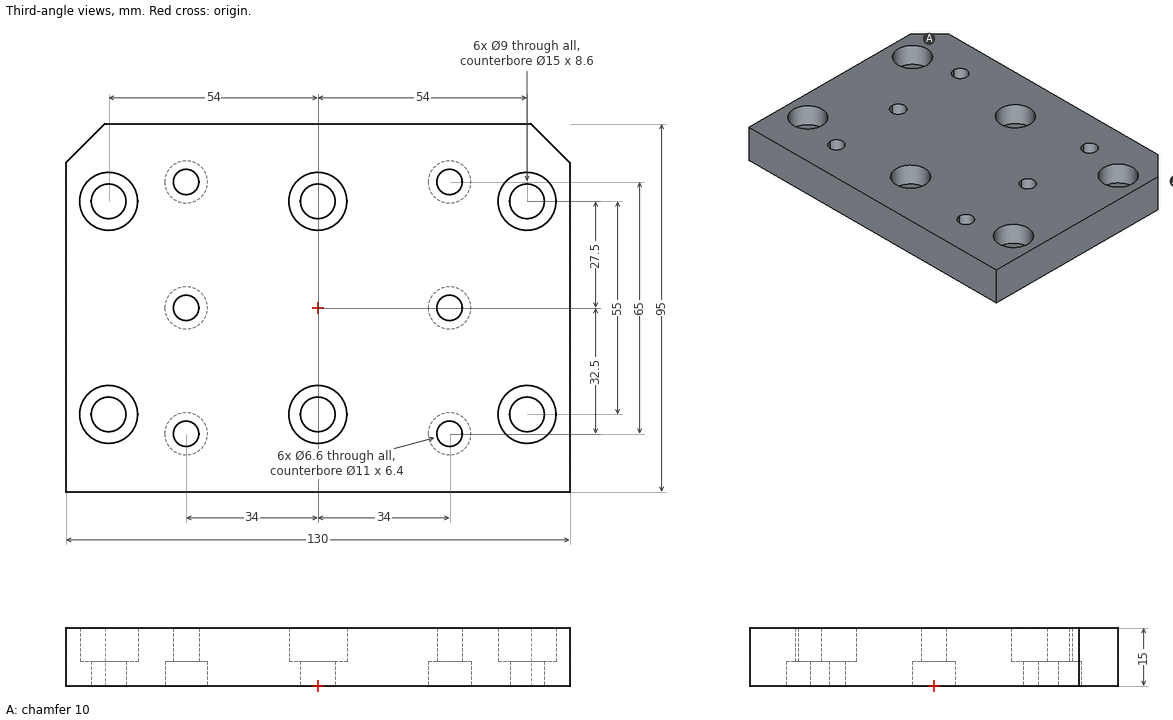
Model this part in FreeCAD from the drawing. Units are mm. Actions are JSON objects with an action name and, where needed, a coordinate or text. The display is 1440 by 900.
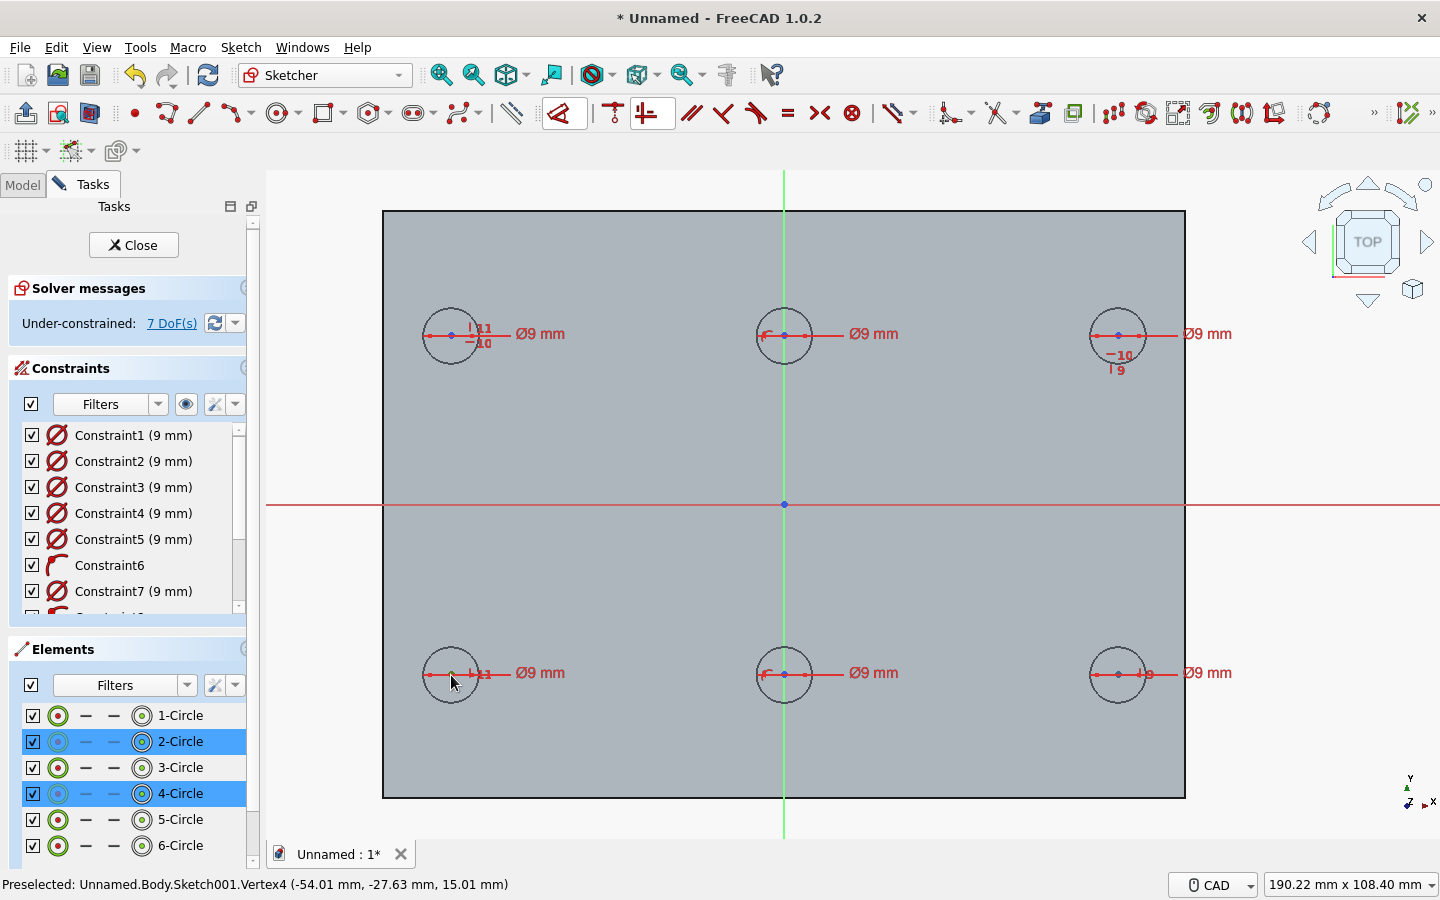
{"action": "key", "text": "h"}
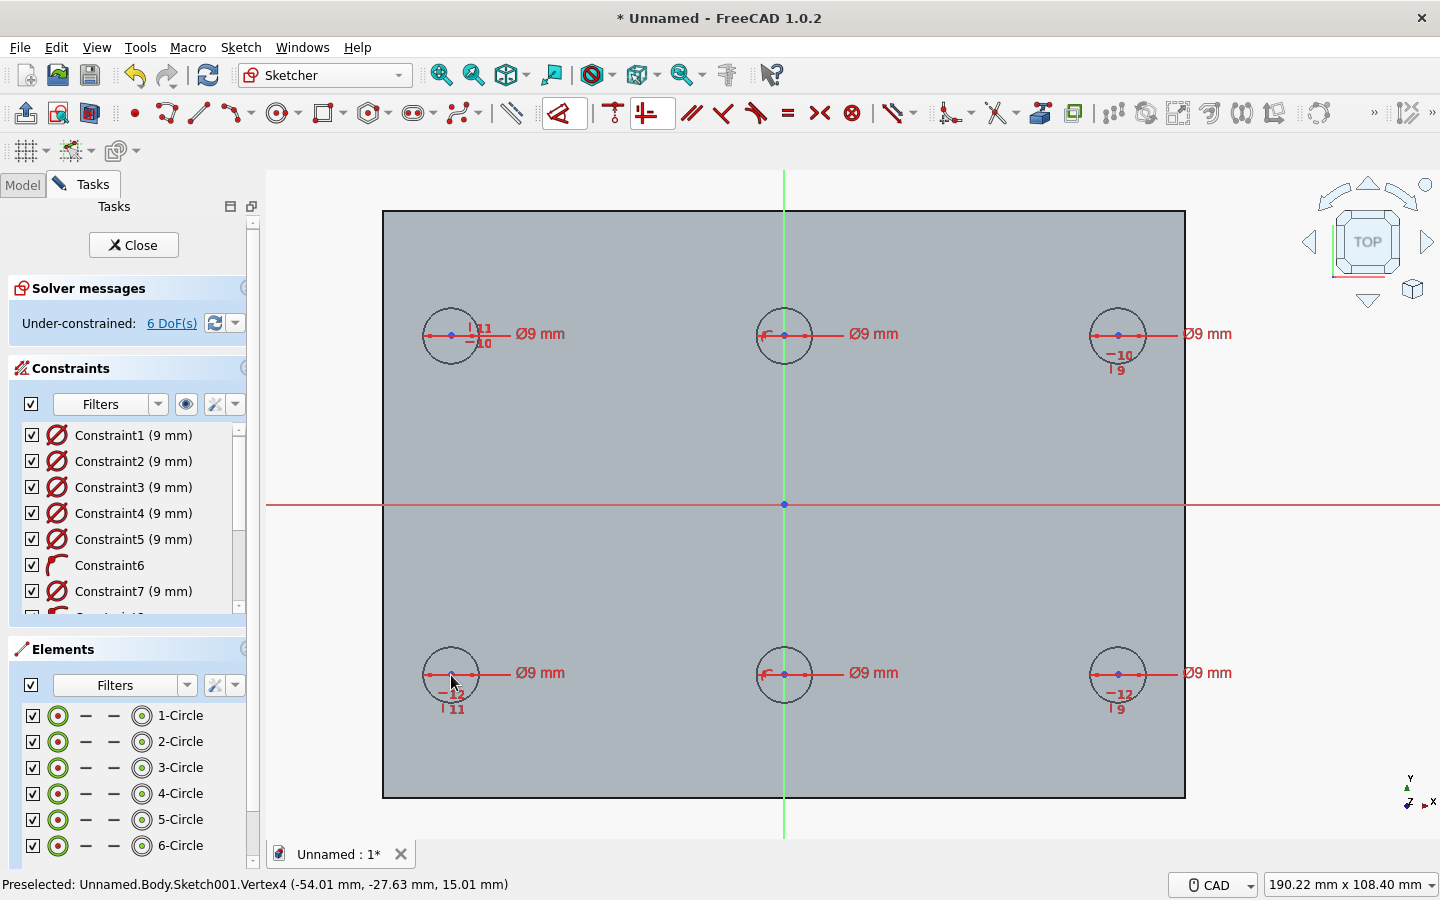
{"action": "left_click", "coordinate": [1118, 336]}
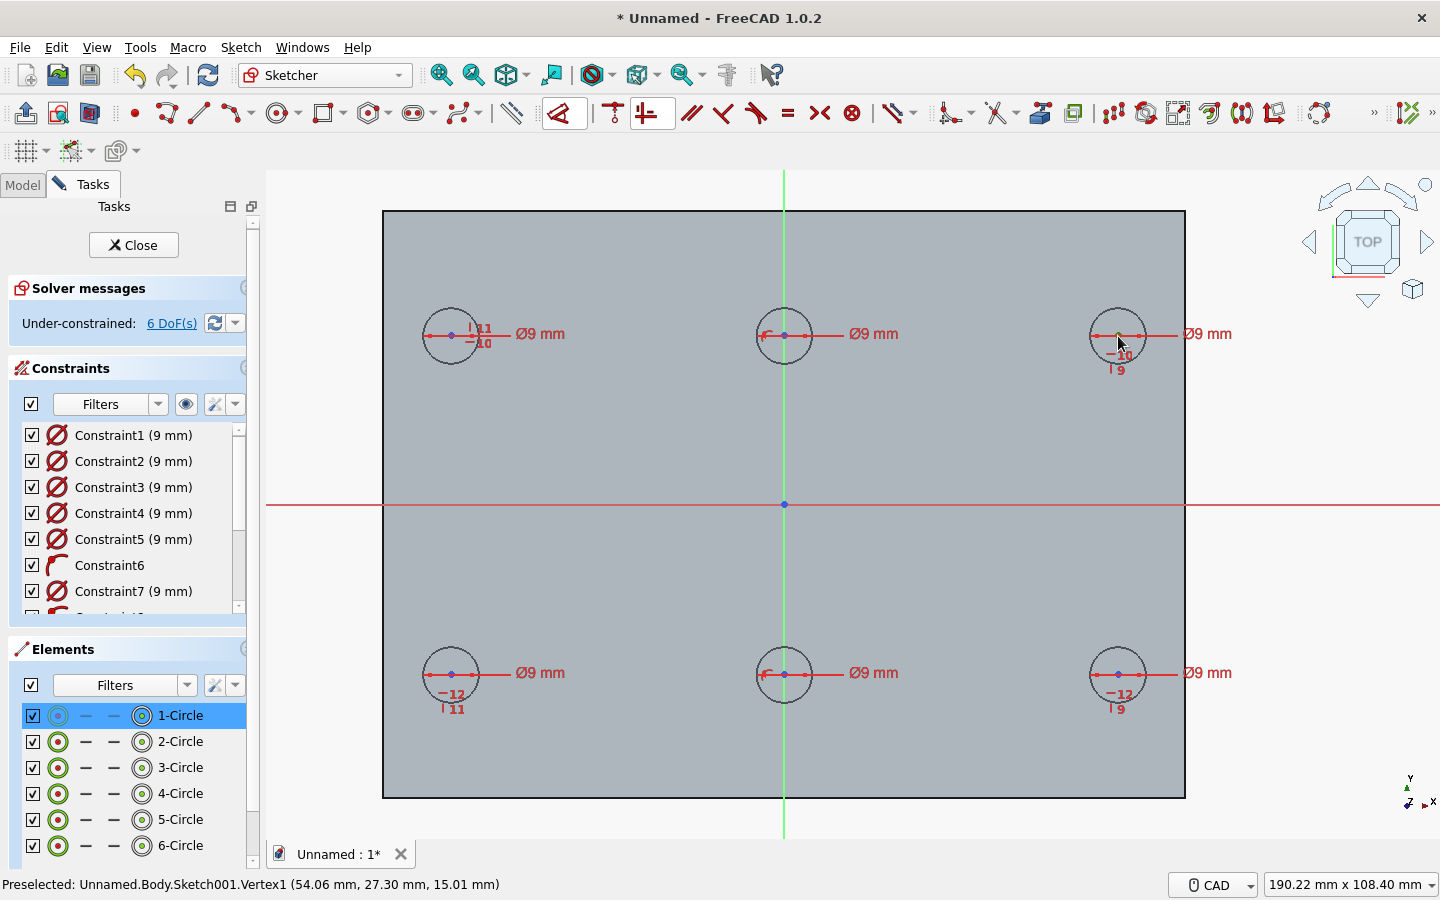
{"action": "left_click", "coordinate": [784, 336]}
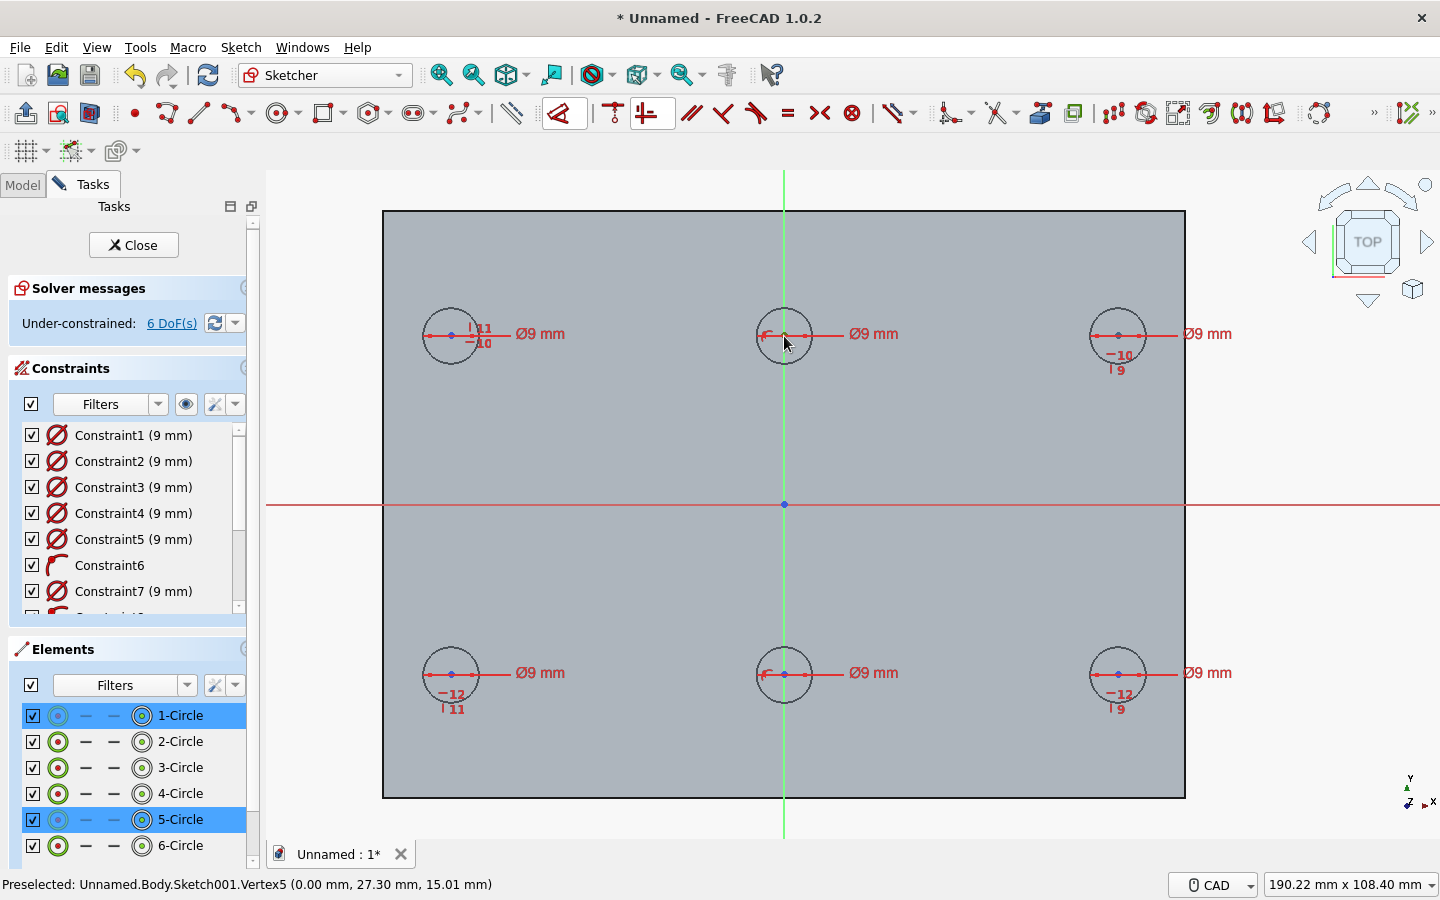
{"action": "key", "text": "h"}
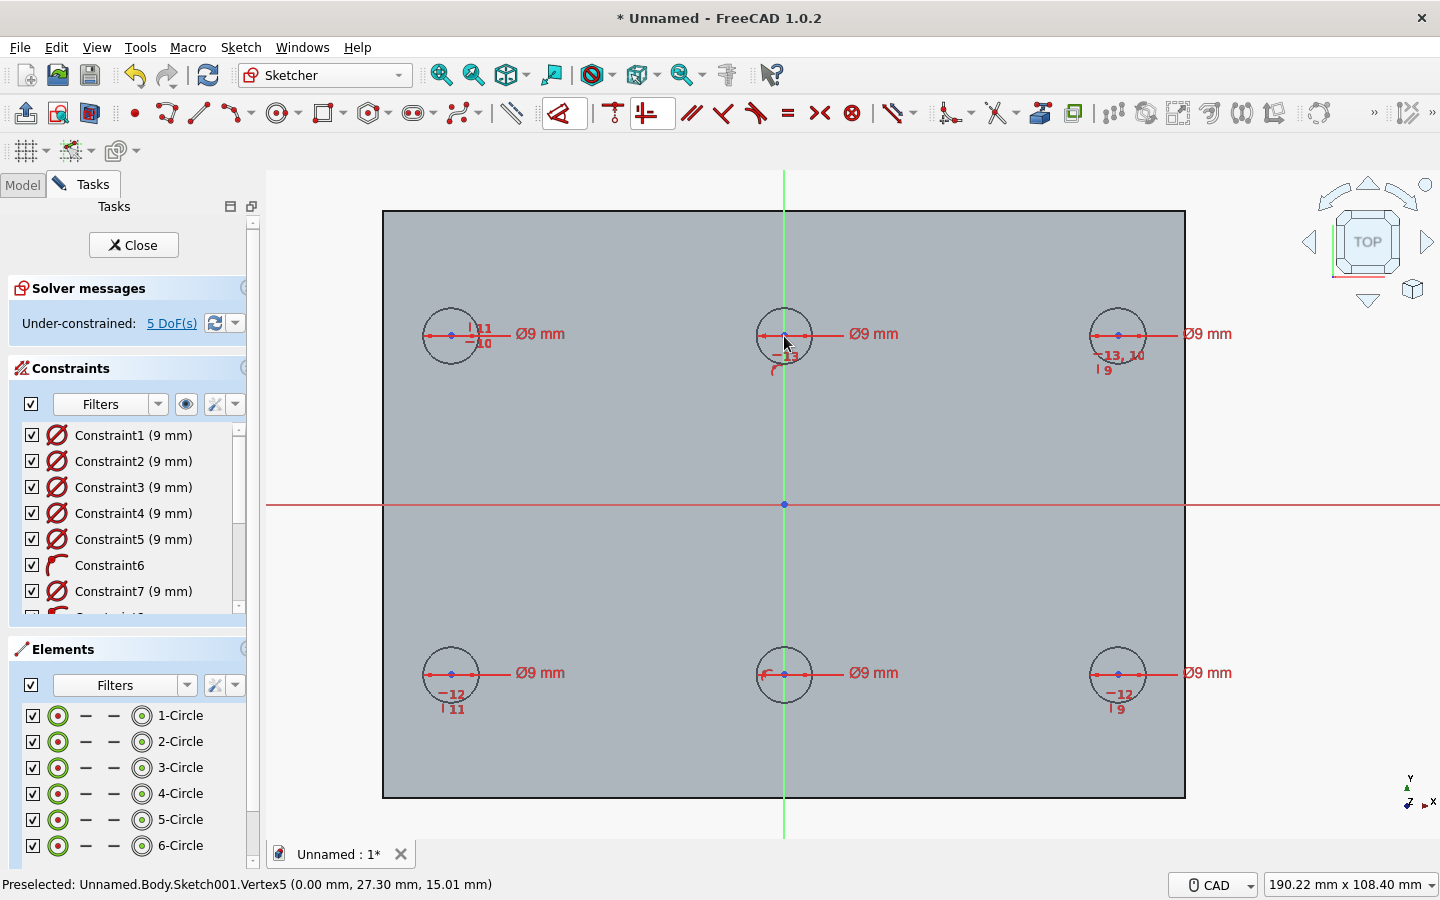
{"action": "left_click", "coordinate": [1118, 675]}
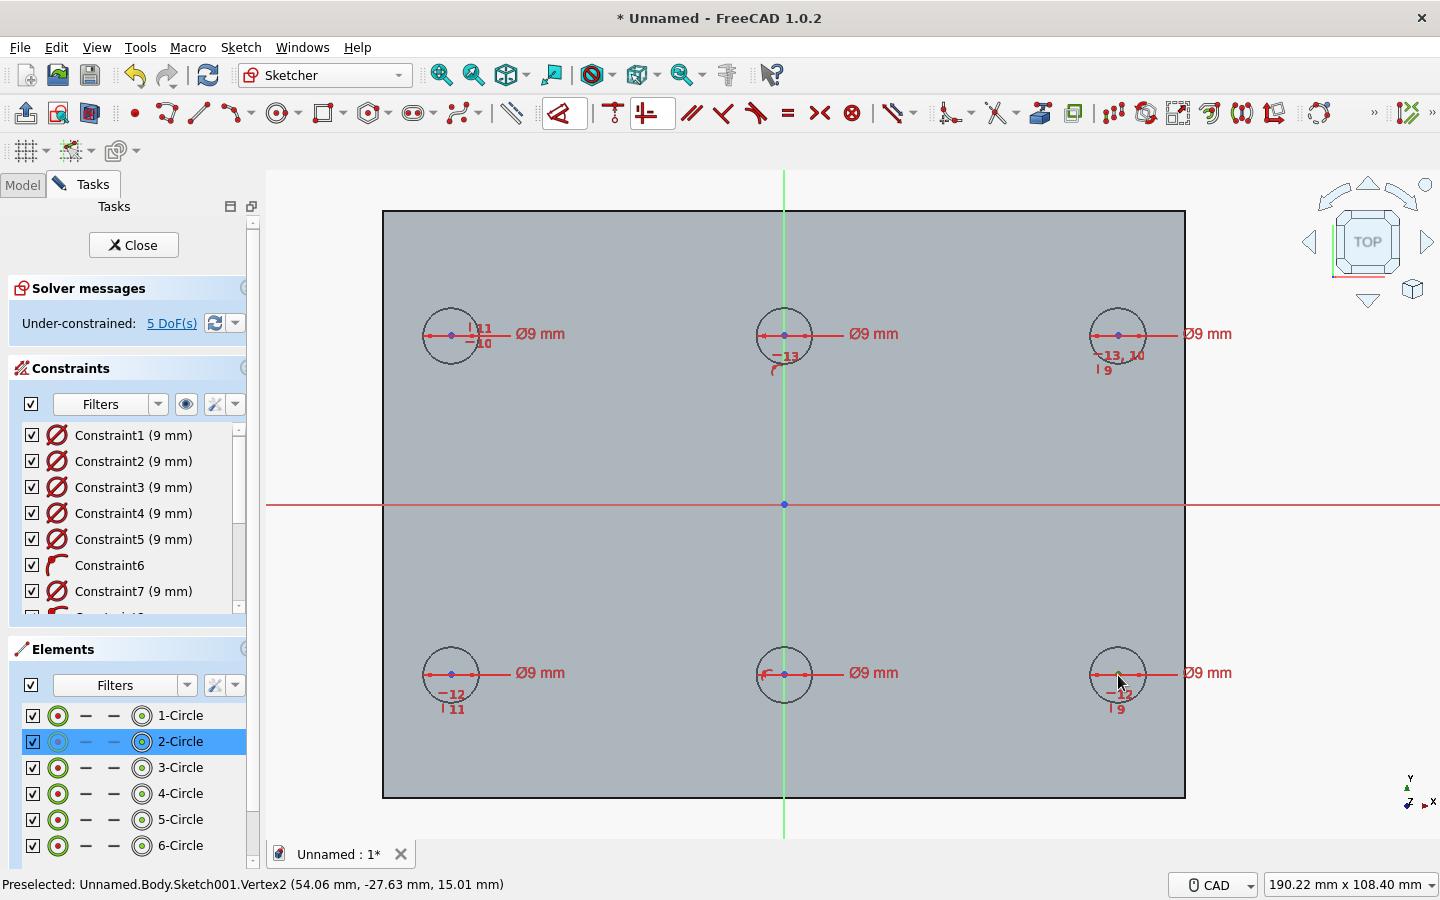
{"action": "left_click", "coordinate": [784, 675]}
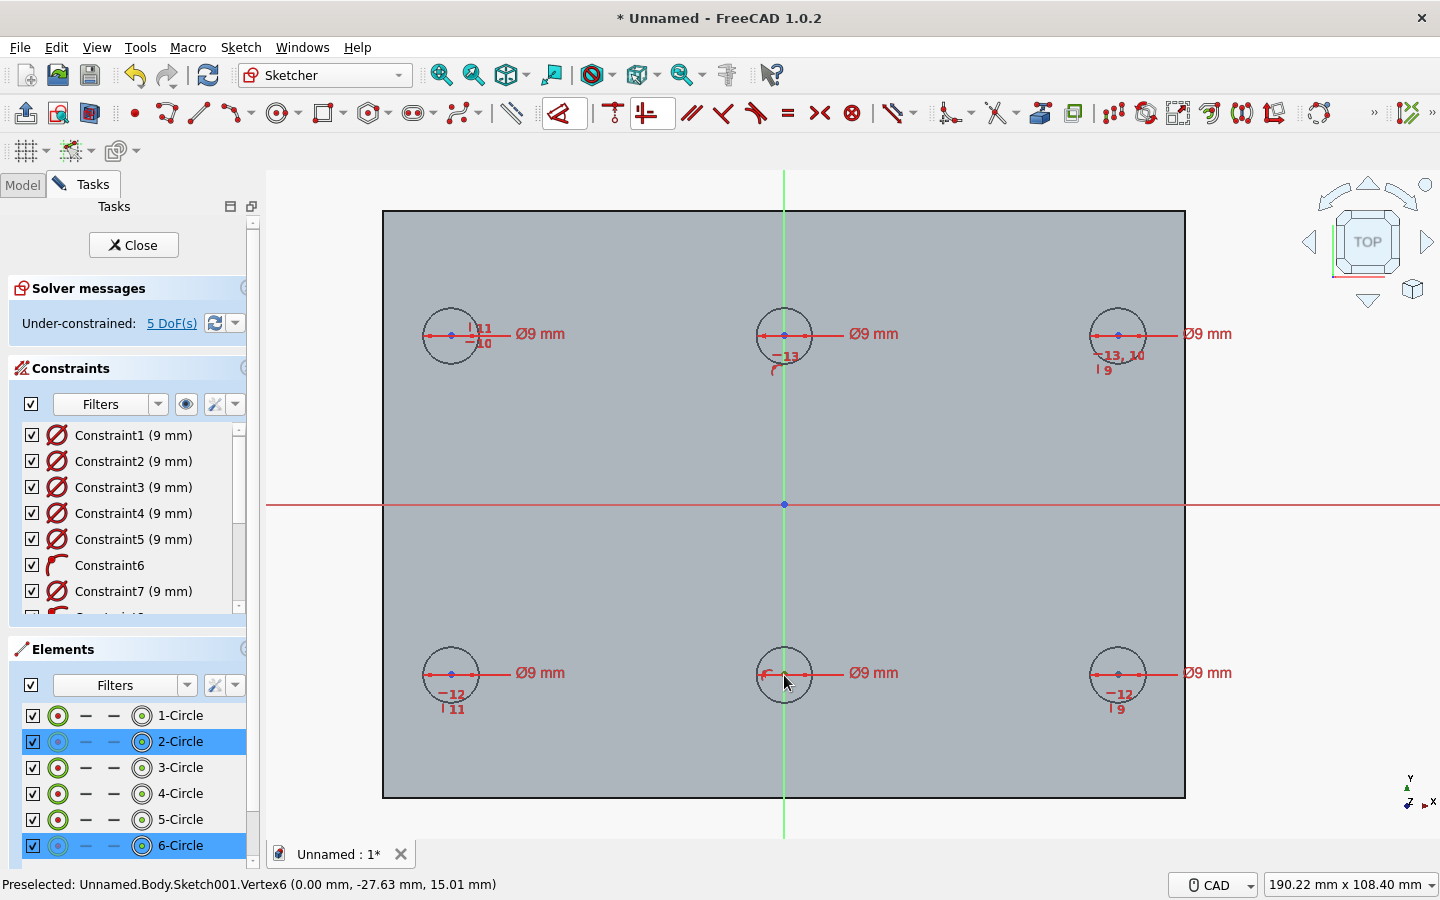
{"action": "key", "text": "h"}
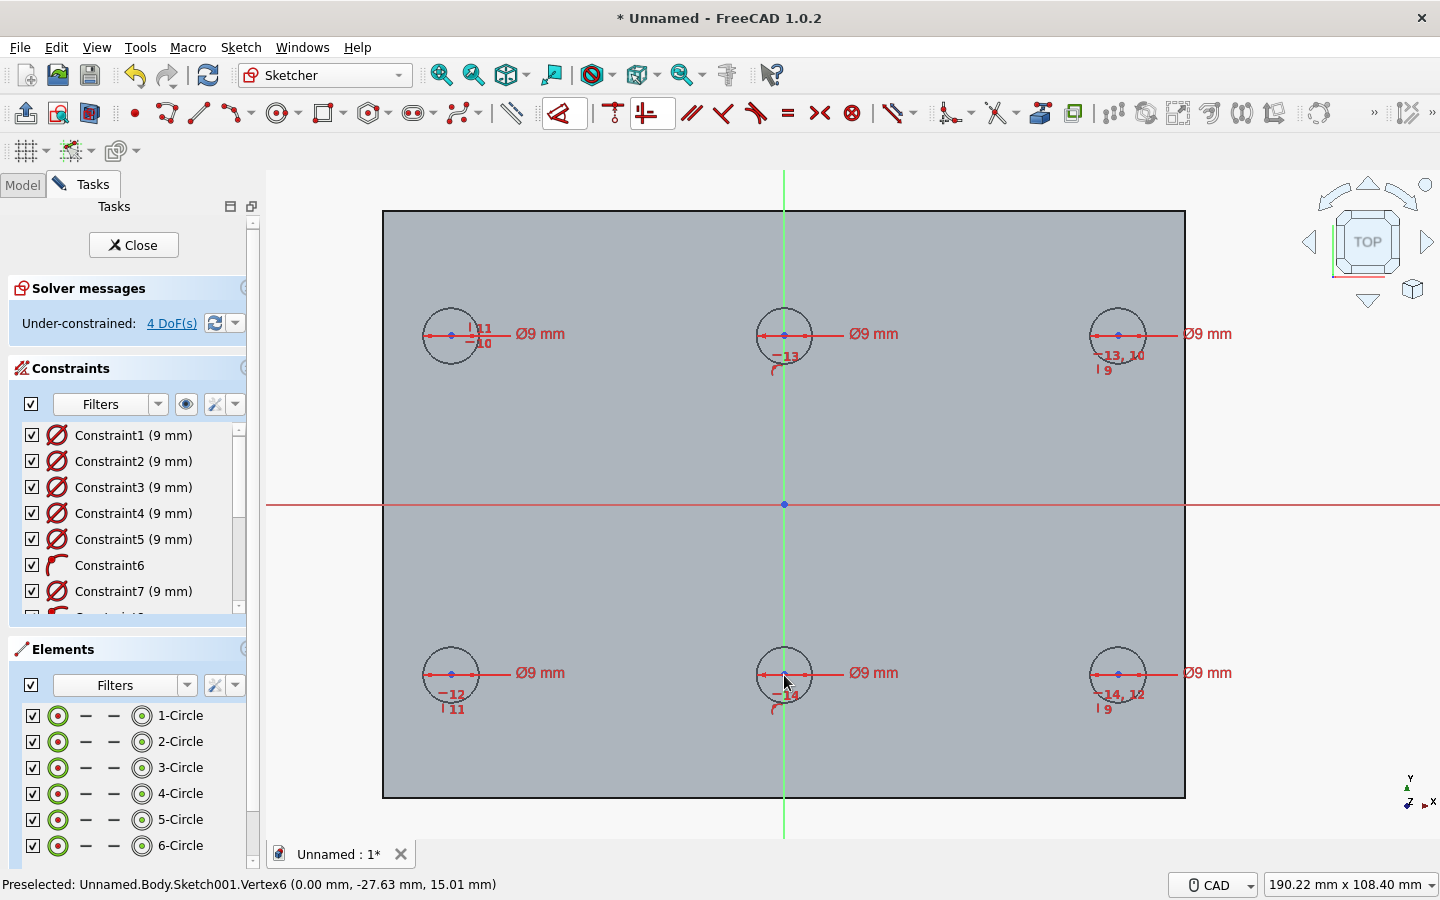
{"action": "key", "text": "d"}